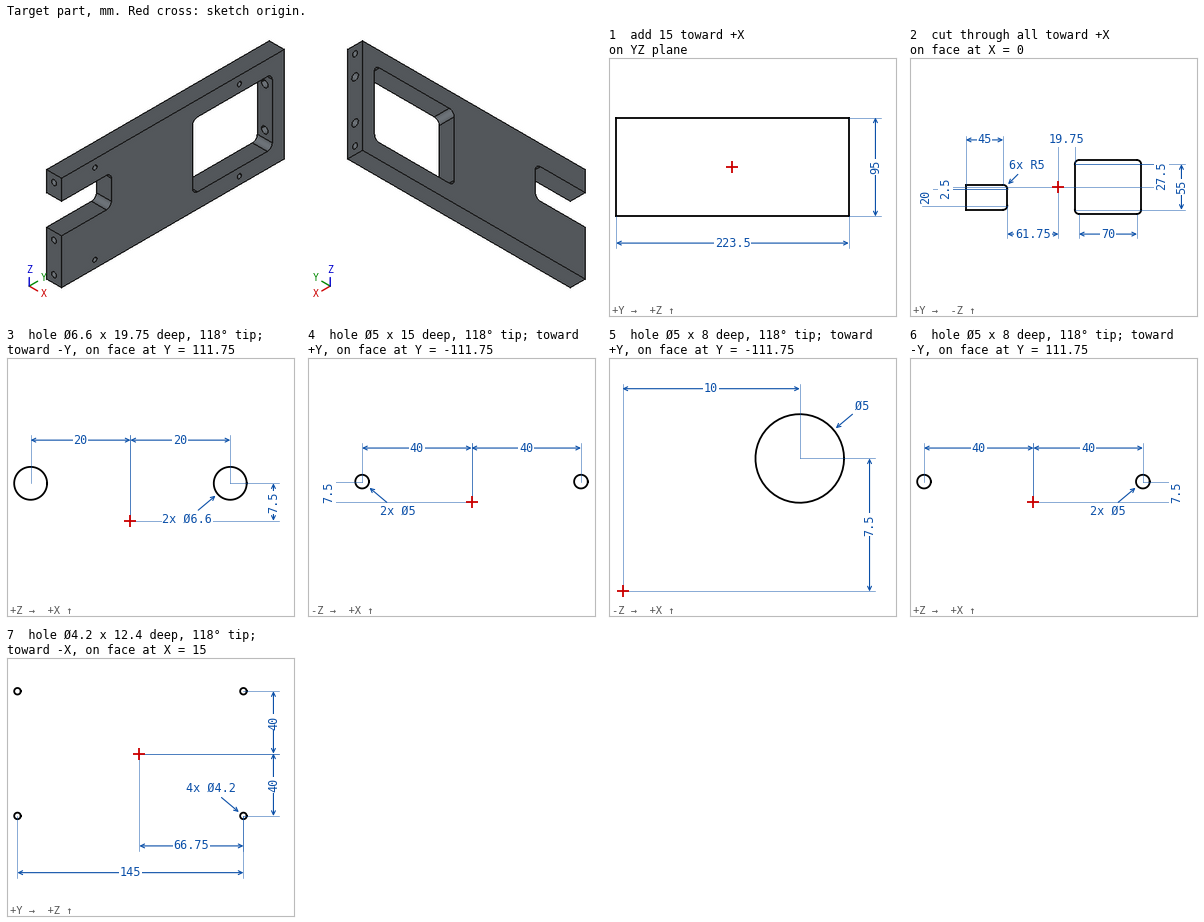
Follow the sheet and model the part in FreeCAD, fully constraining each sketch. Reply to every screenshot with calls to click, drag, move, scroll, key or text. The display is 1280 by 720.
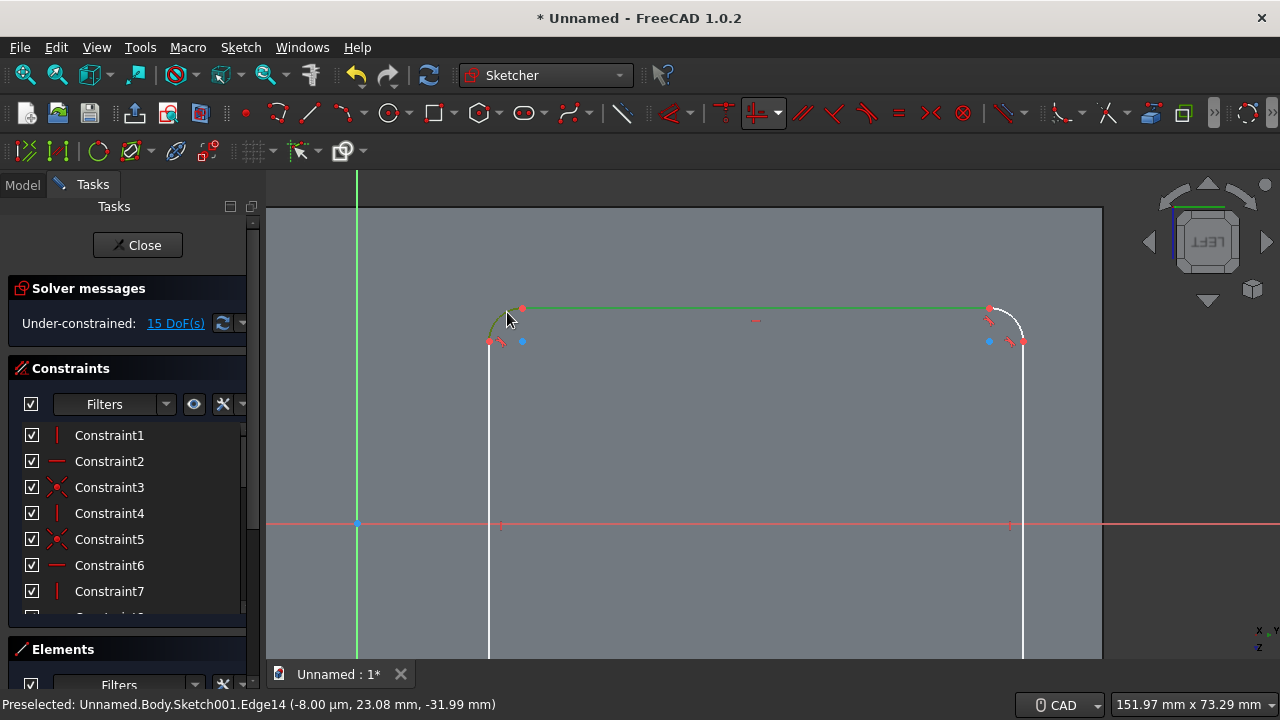
click(868, 114)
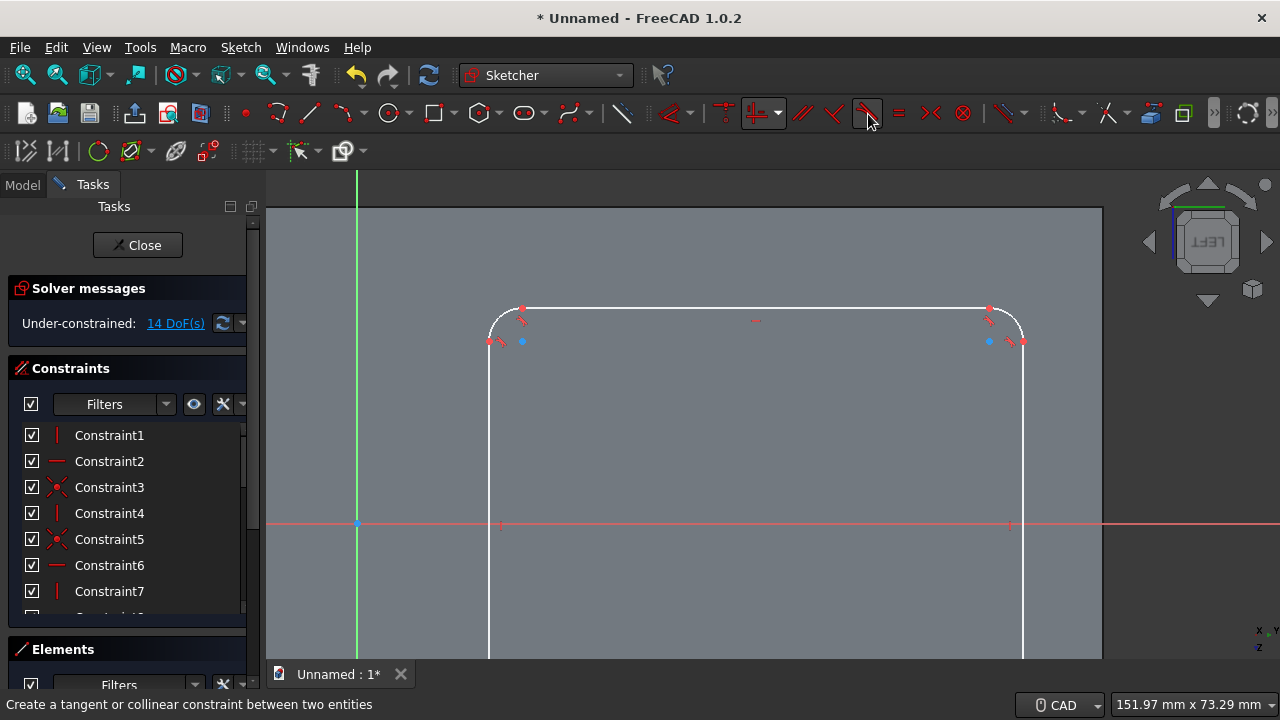
scroll(1021, 325, down, 4)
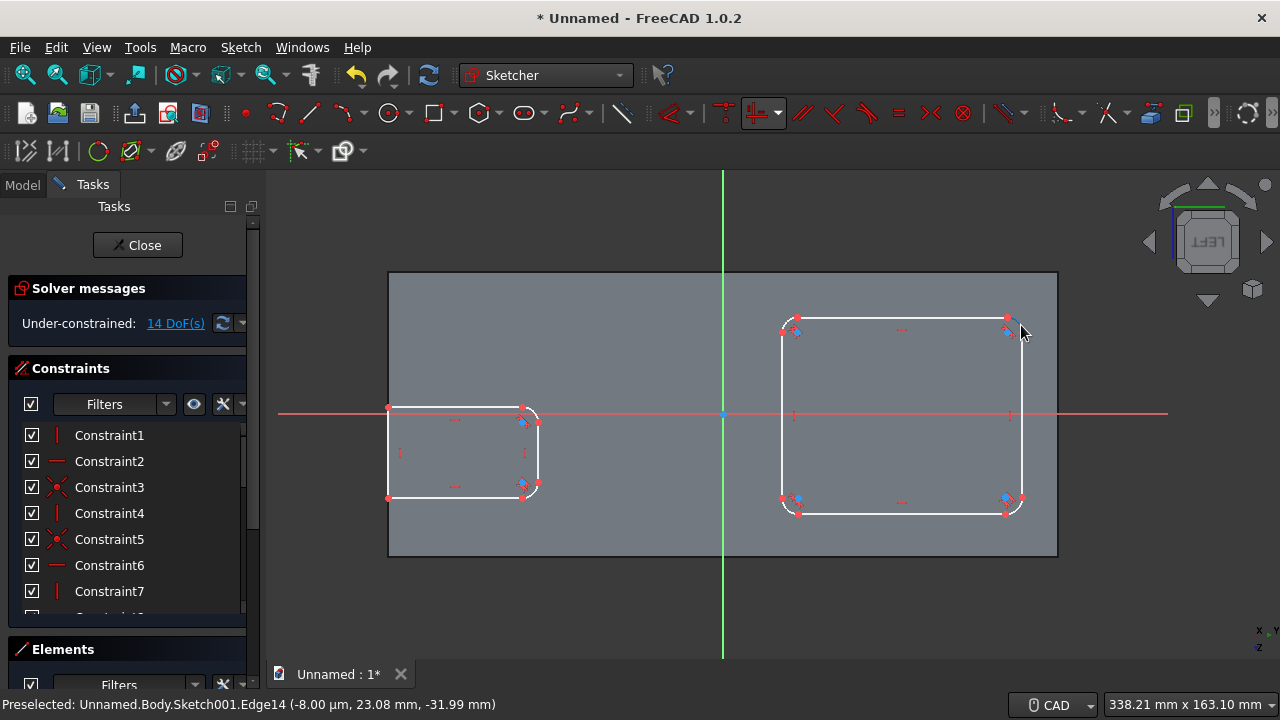
scroll(536, 415, up, 4)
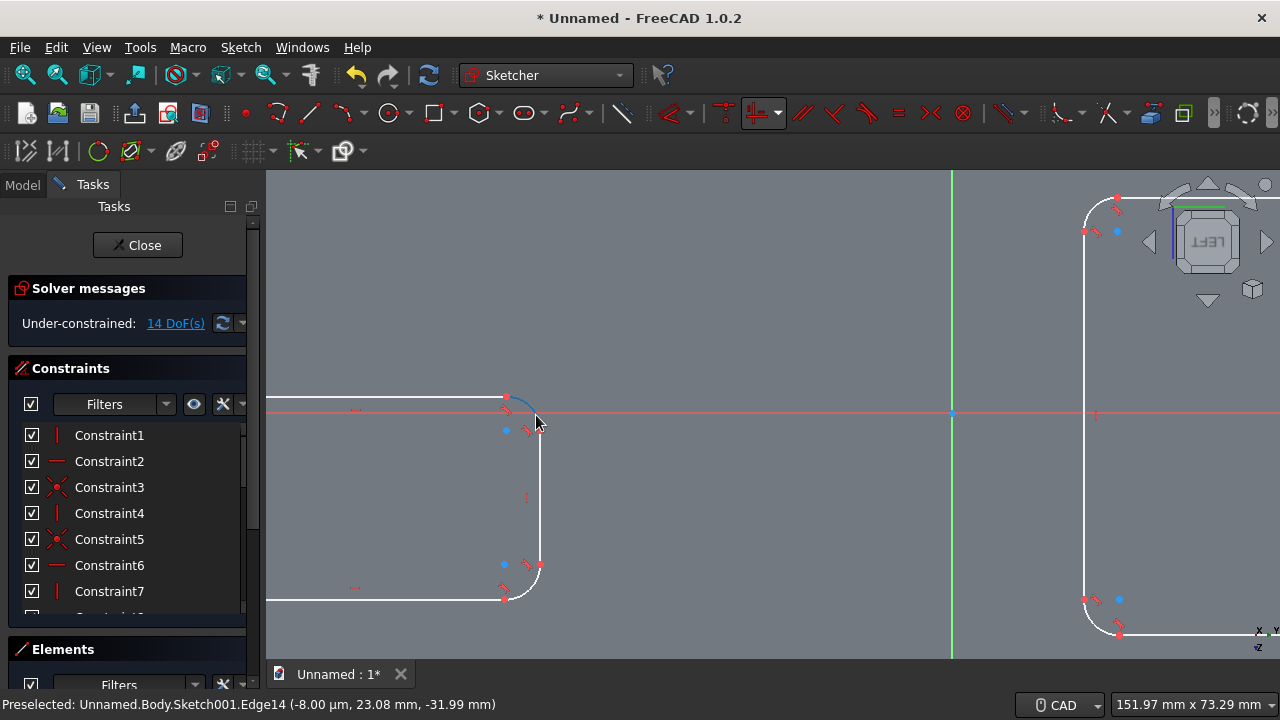
click(537, 415)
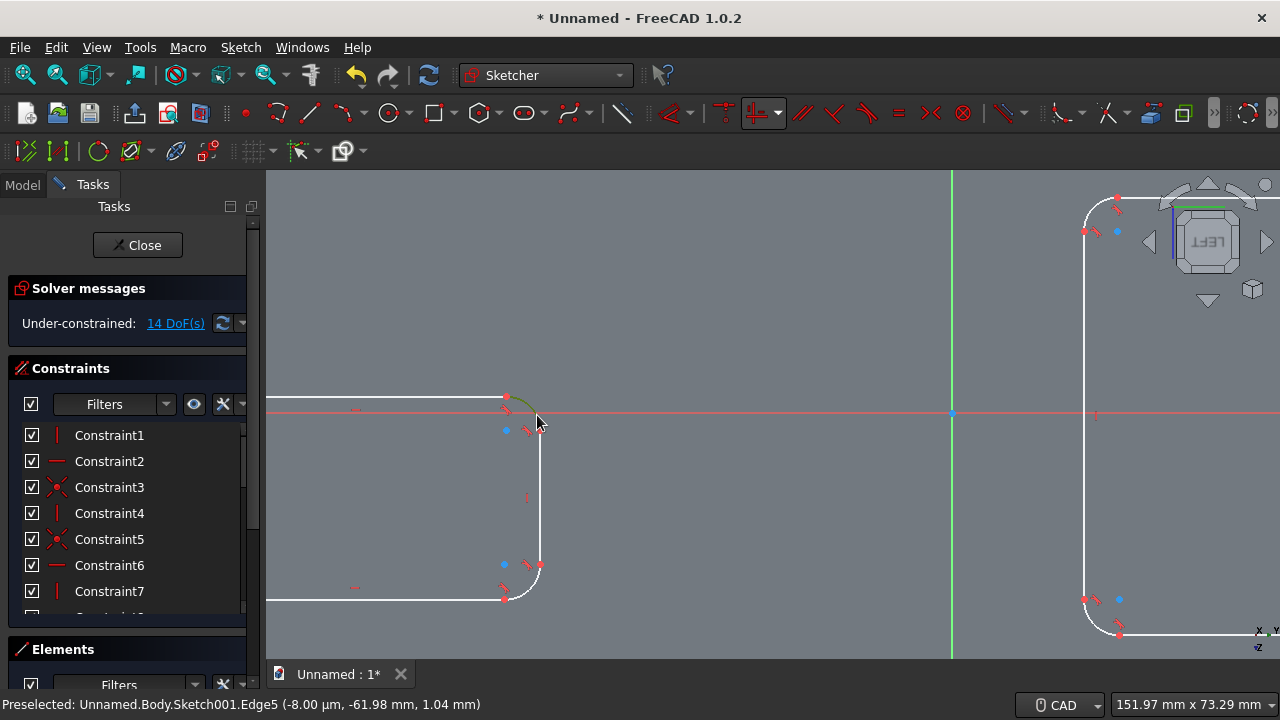
click(521, 596)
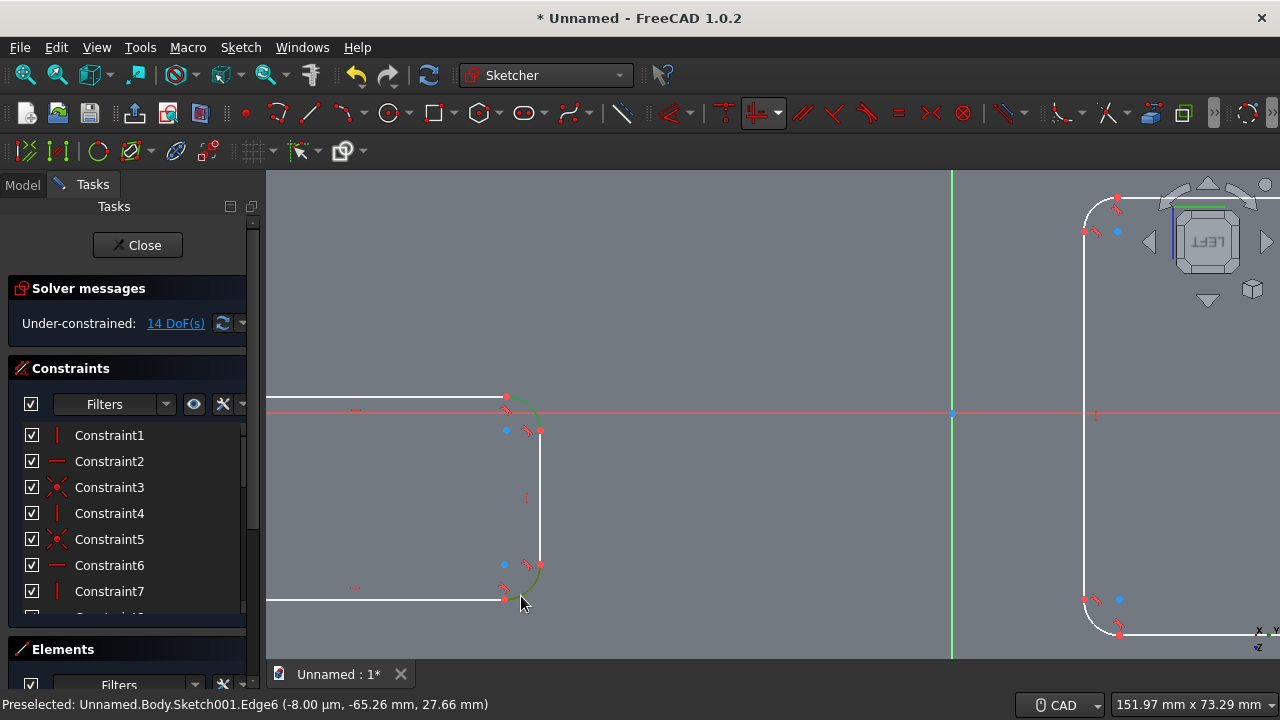
click(1088, 616)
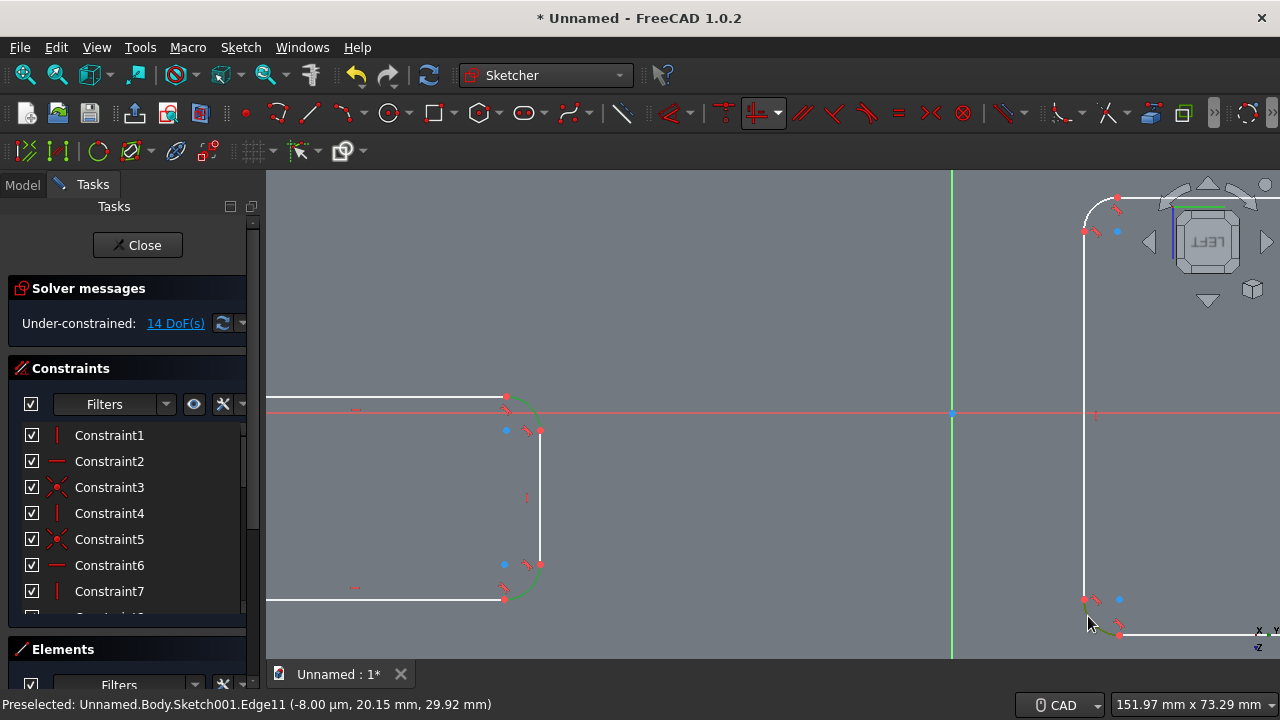
scroll(535, 416, down, 4)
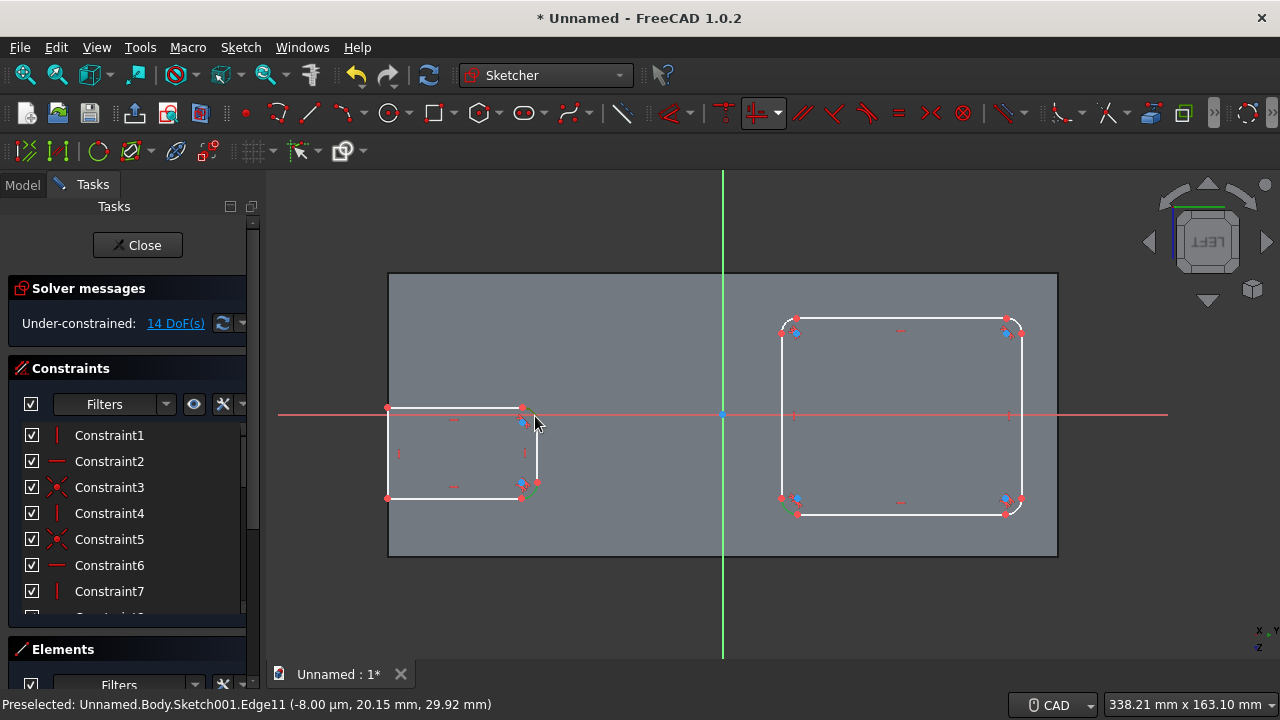
scroll(1013, 513, up, 3)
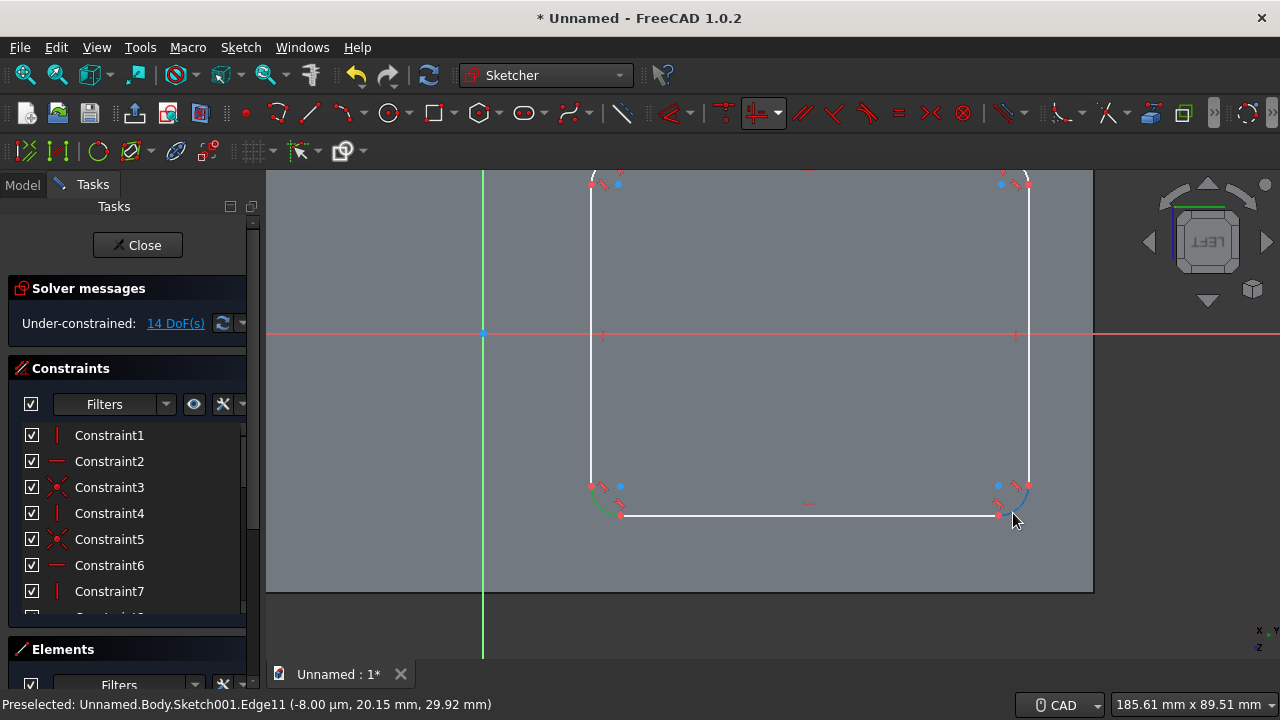
click(1012, 512)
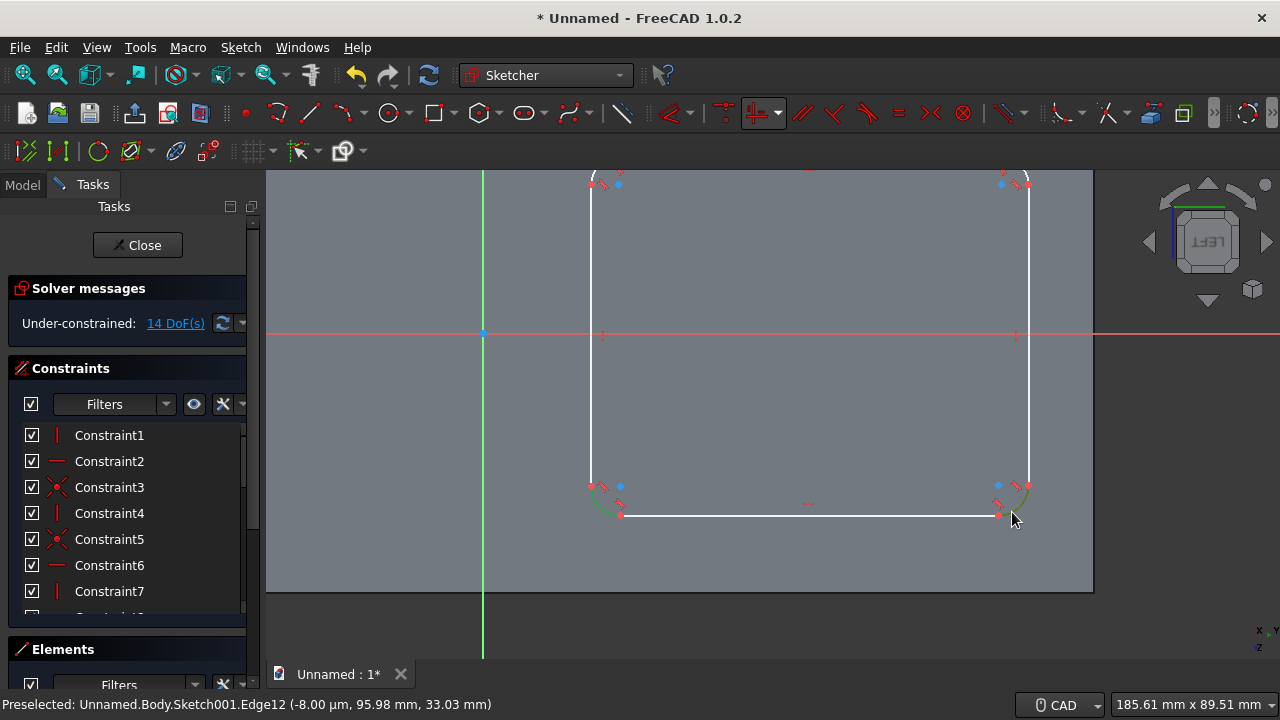
scroll(1014, 513, down, 3)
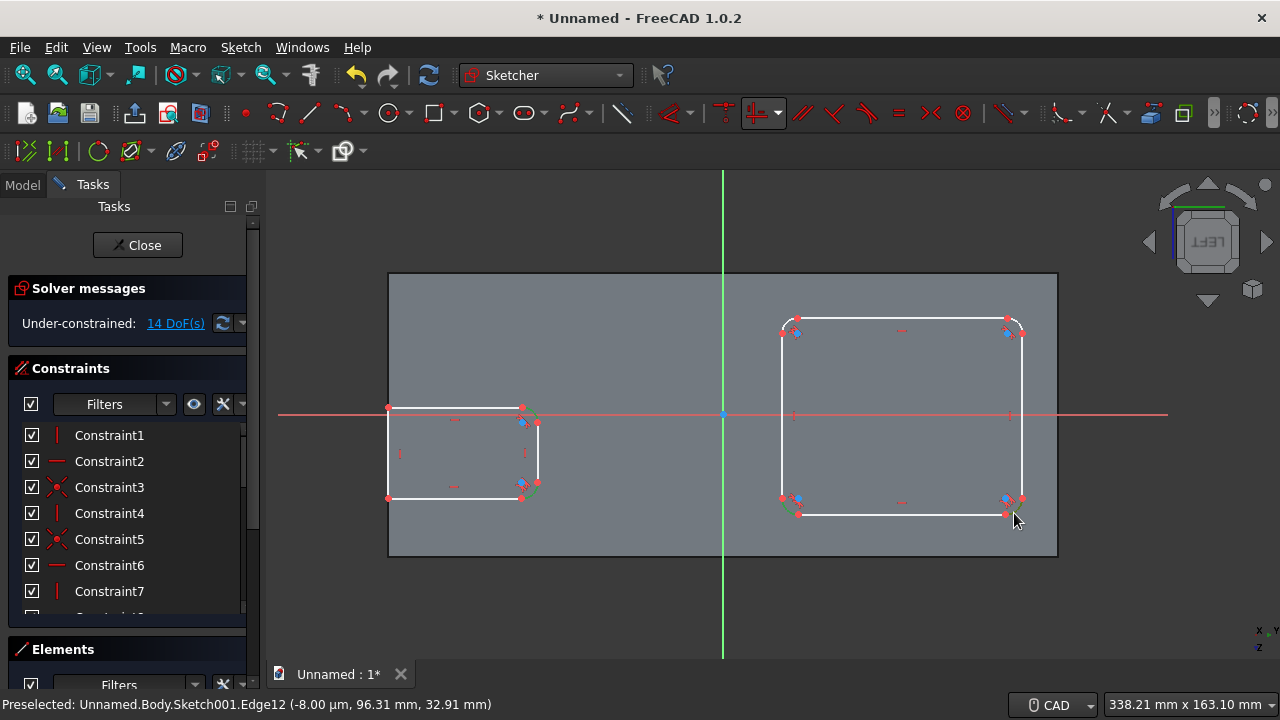
scroll(1021, 326, up, 4)